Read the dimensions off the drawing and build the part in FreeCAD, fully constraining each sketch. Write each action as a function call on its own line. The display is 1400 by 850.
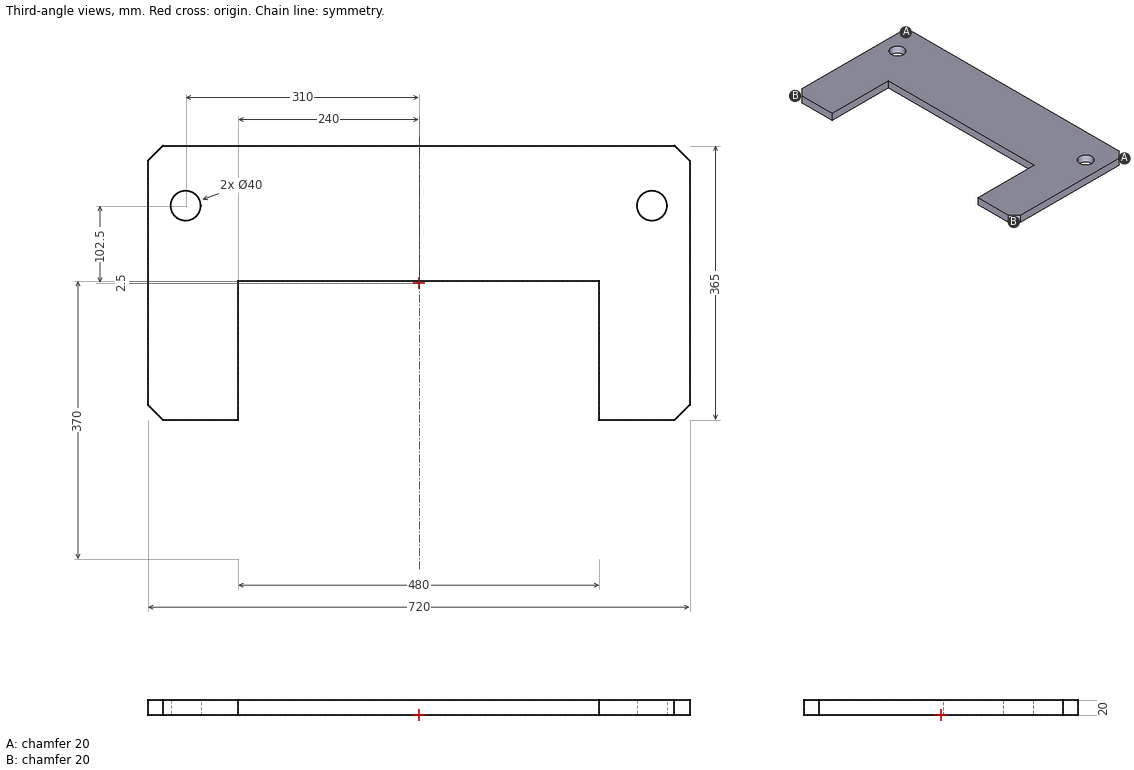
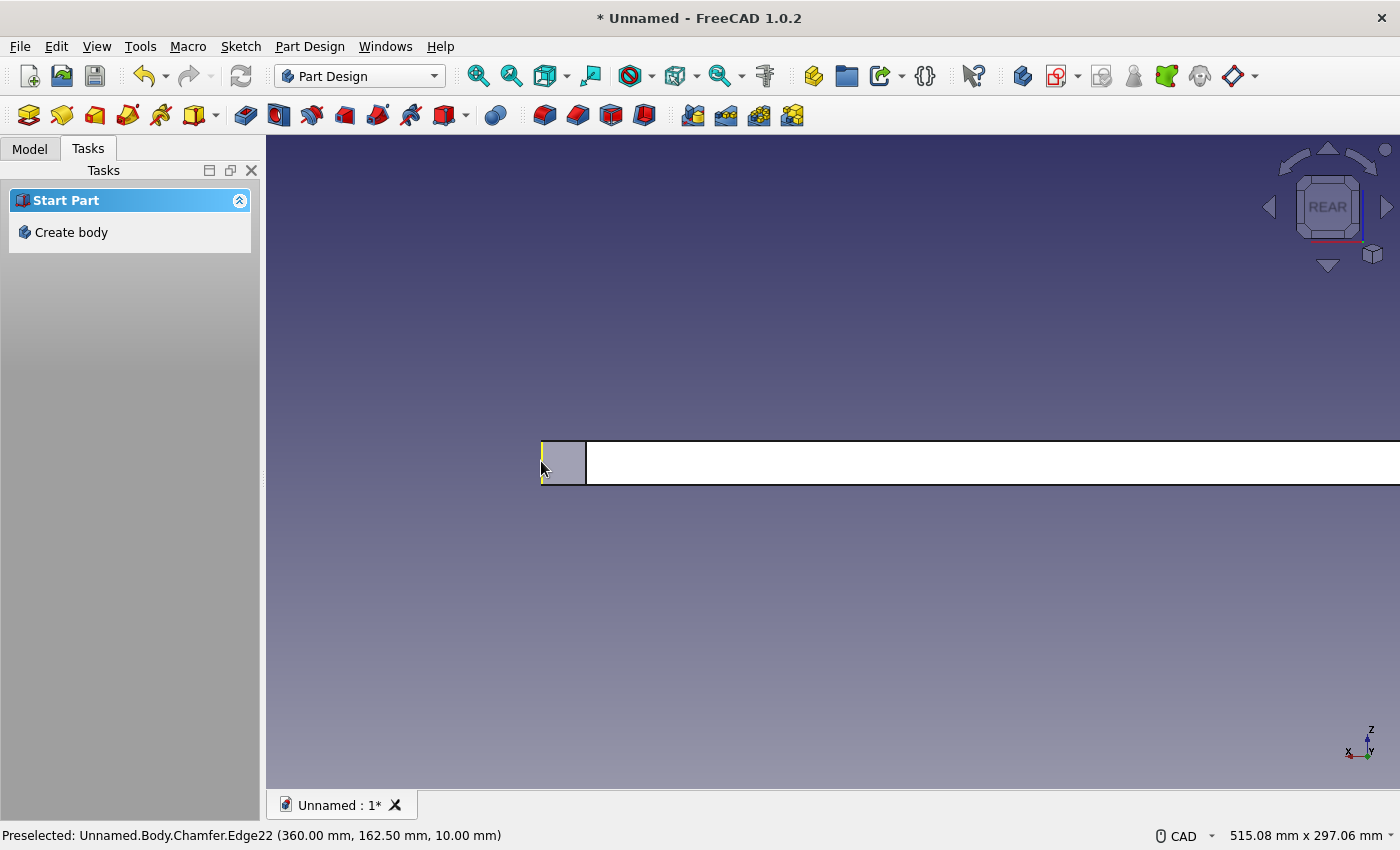
click(479, 76)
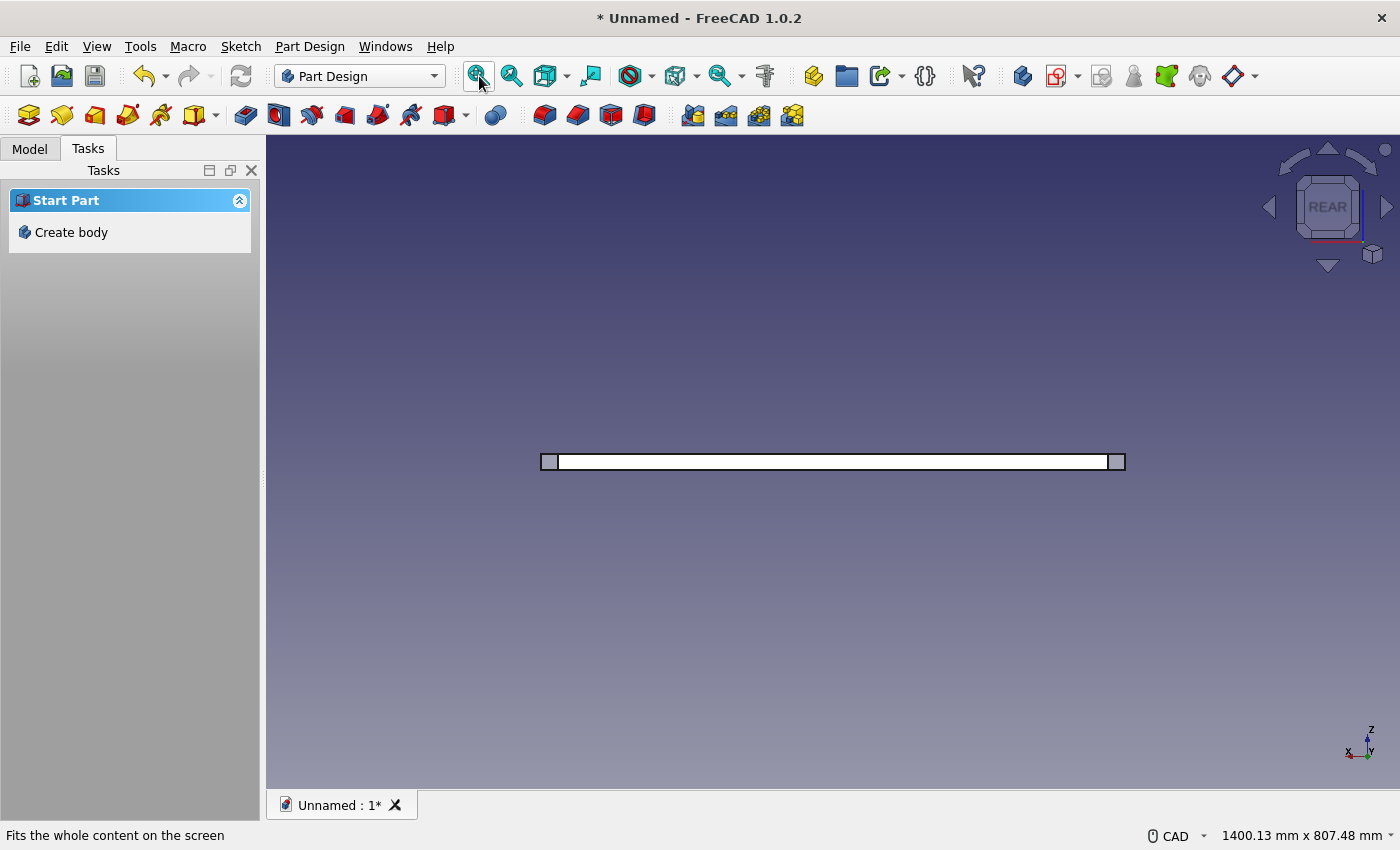
key(0)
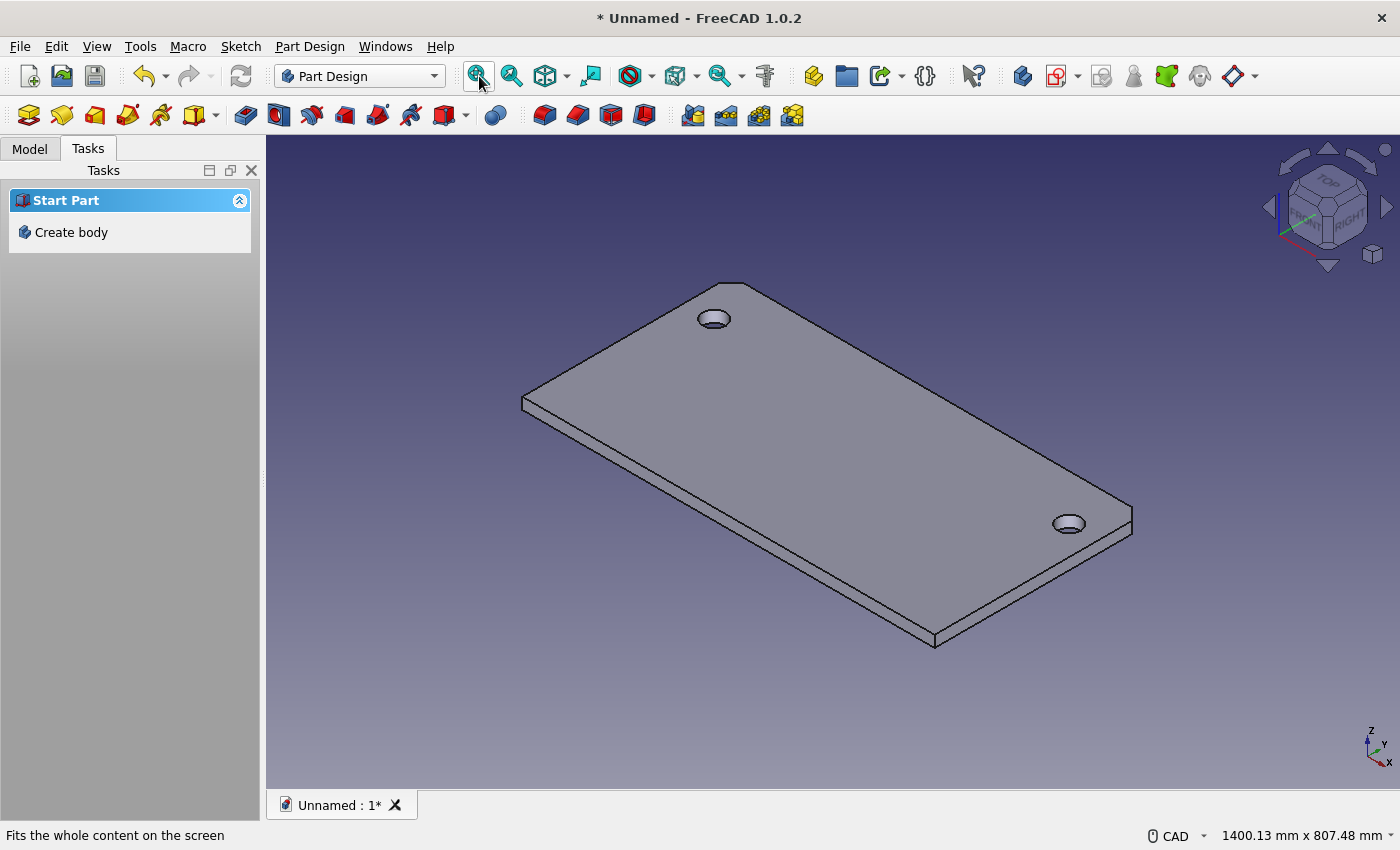
click(935, 640)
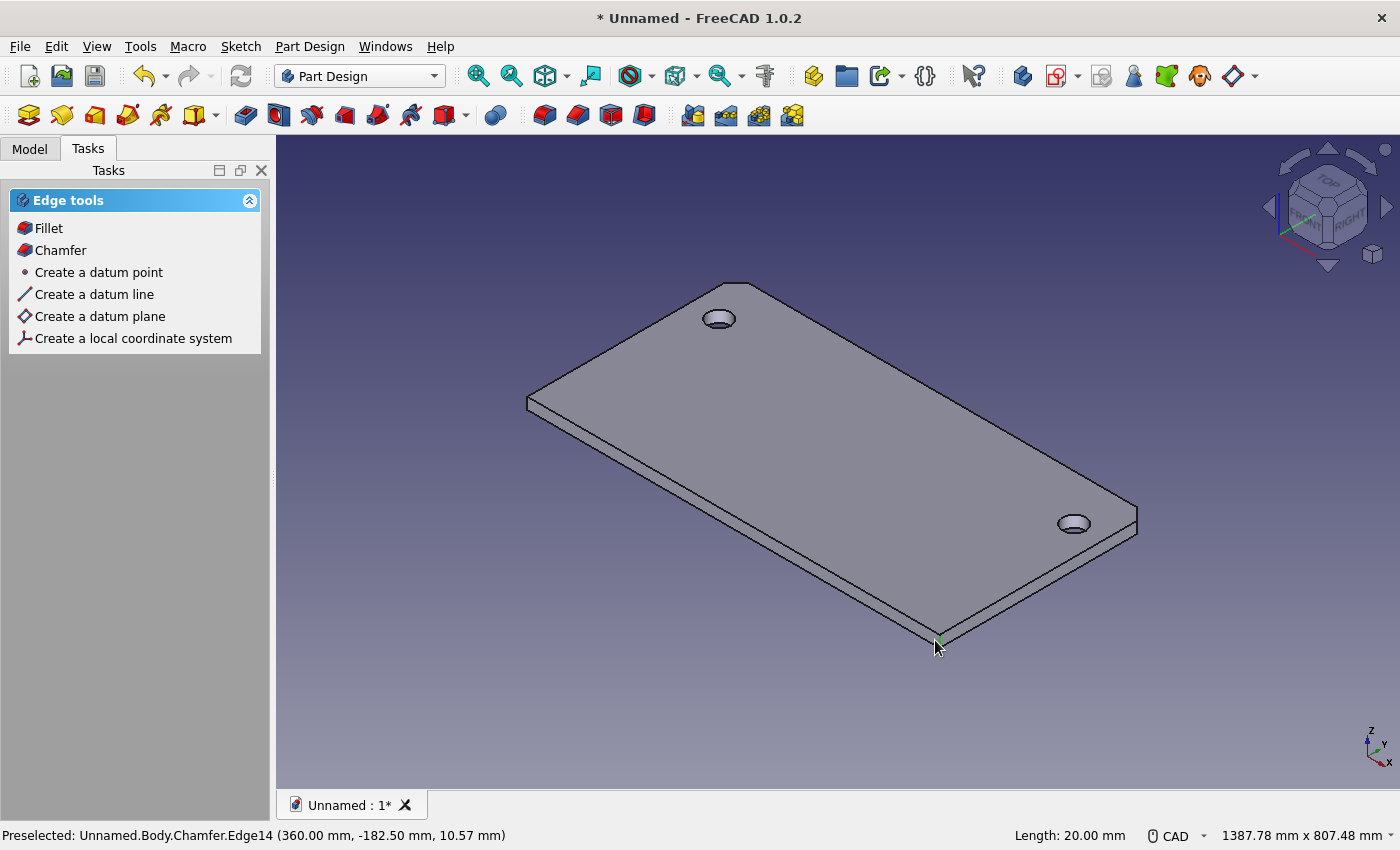
scroll(527, 402, up, 5)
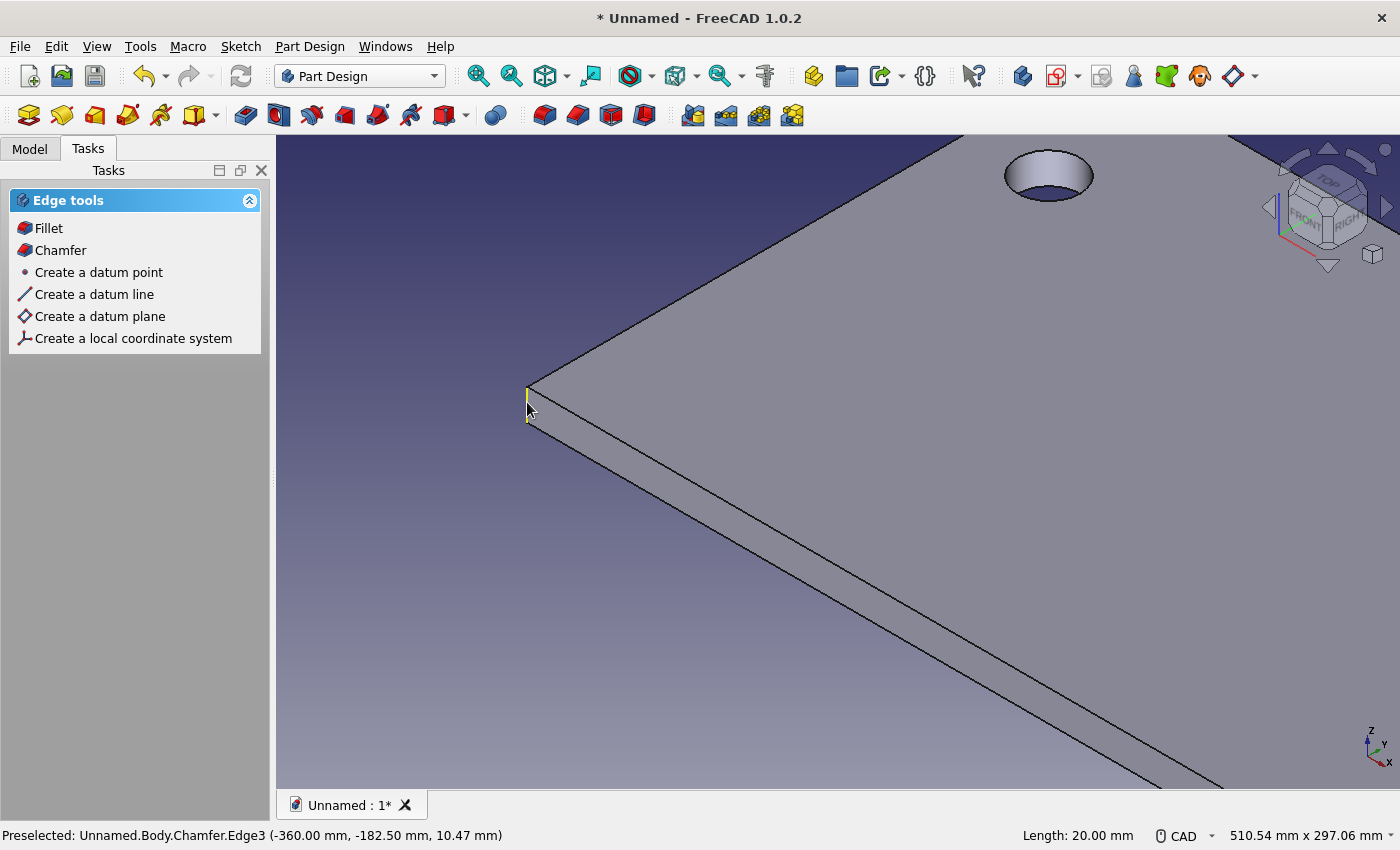
key(v)
key(f)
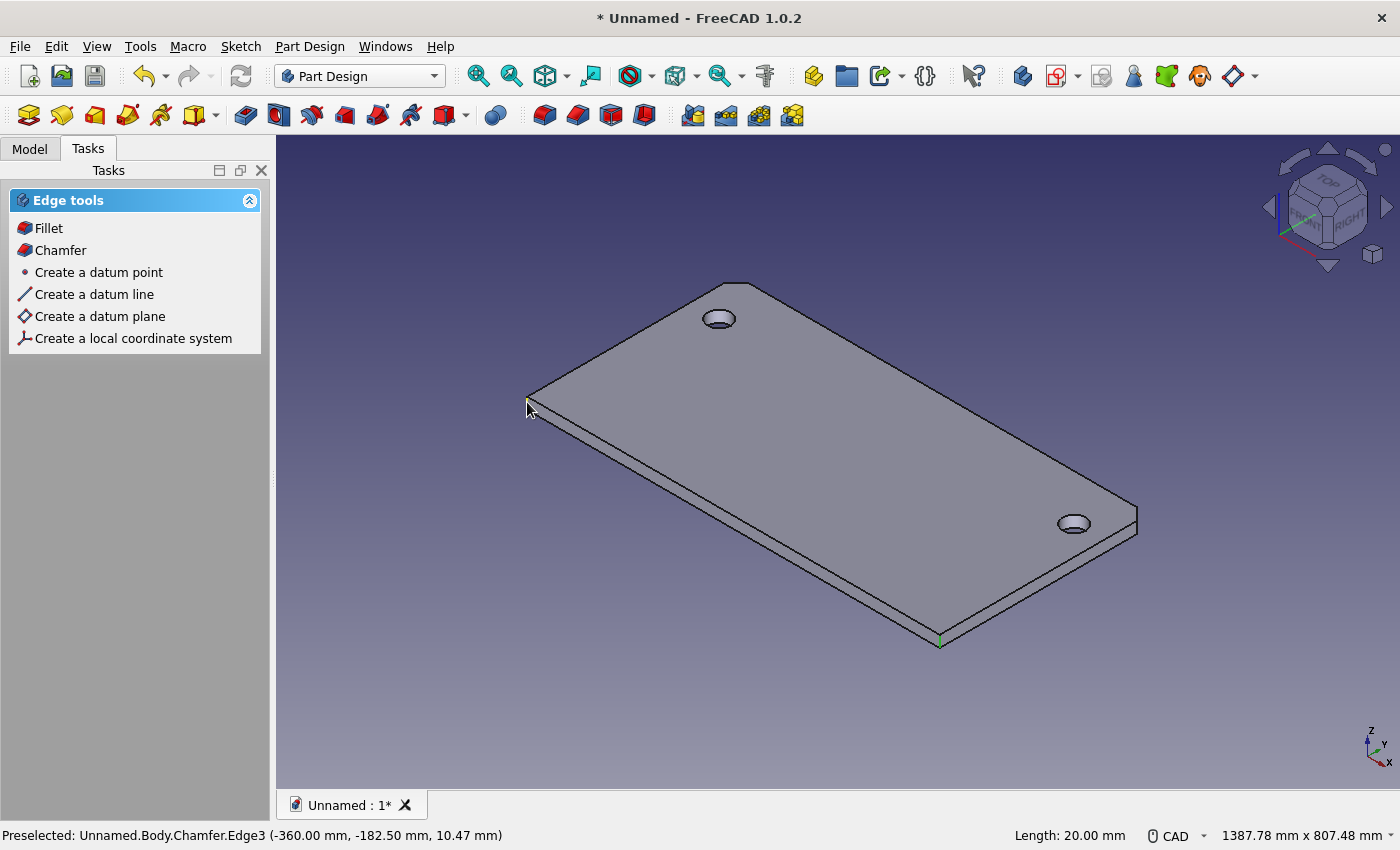
key(2)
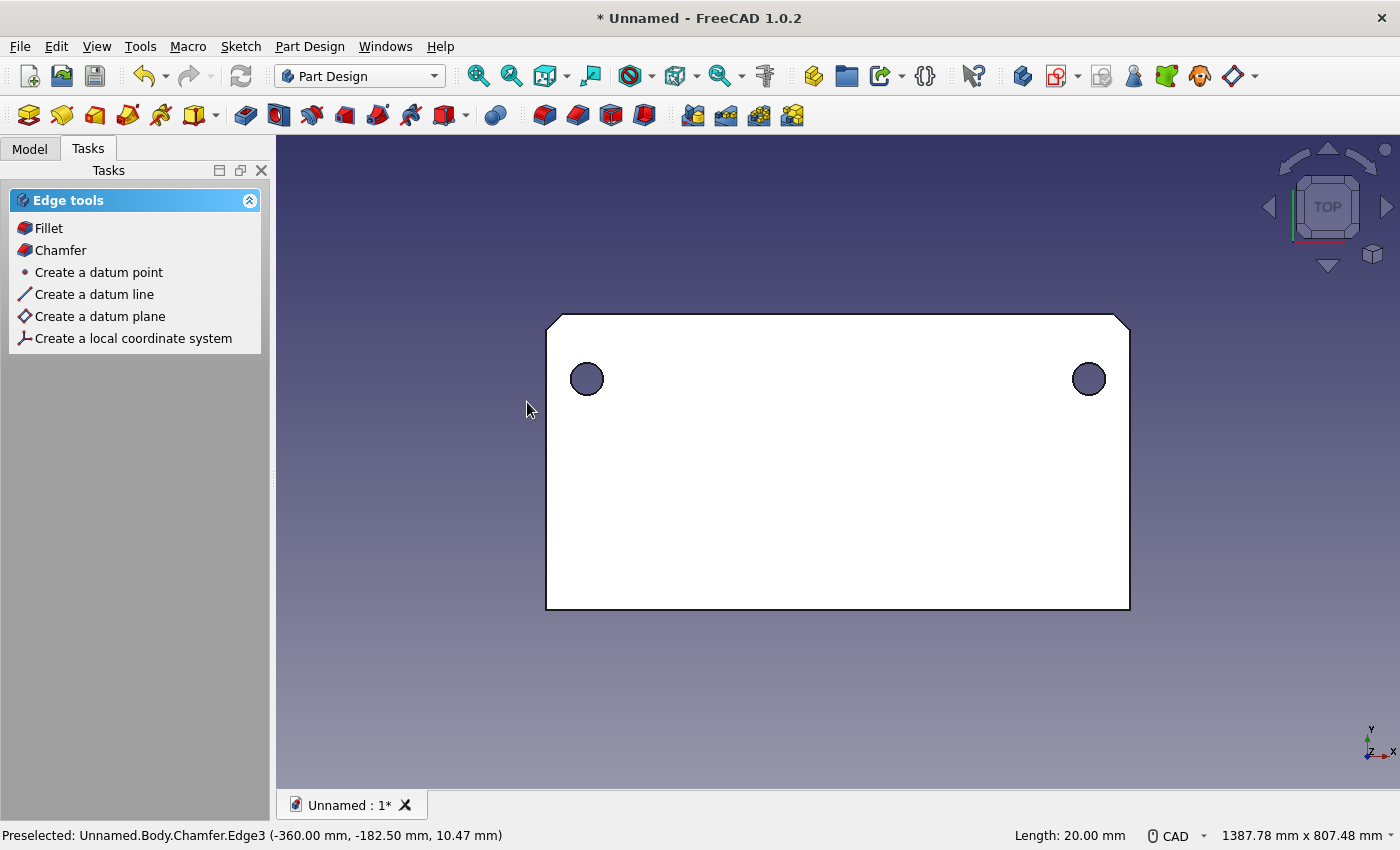
scroll(546, 609, up, 5)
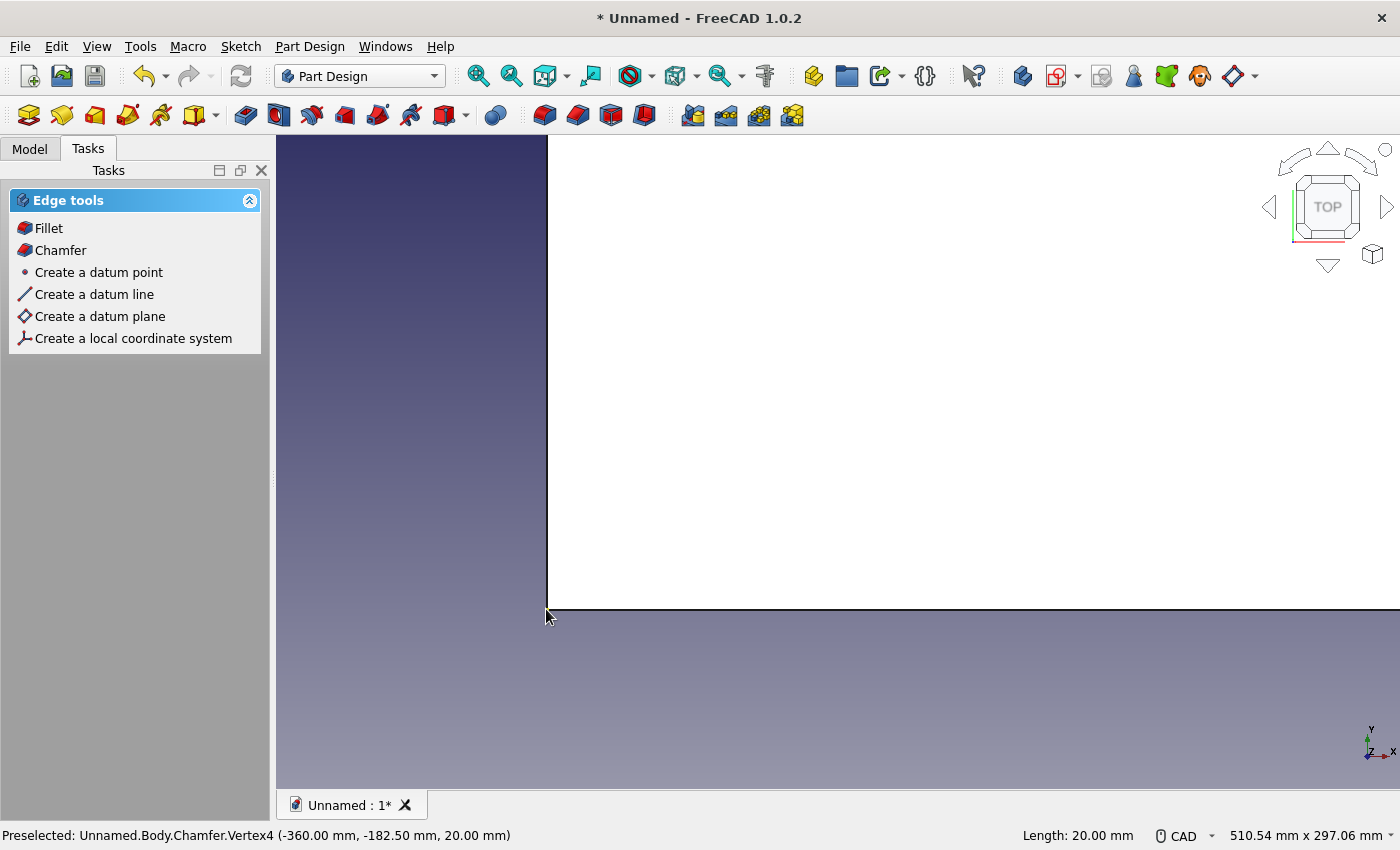
key(v)
key(f)